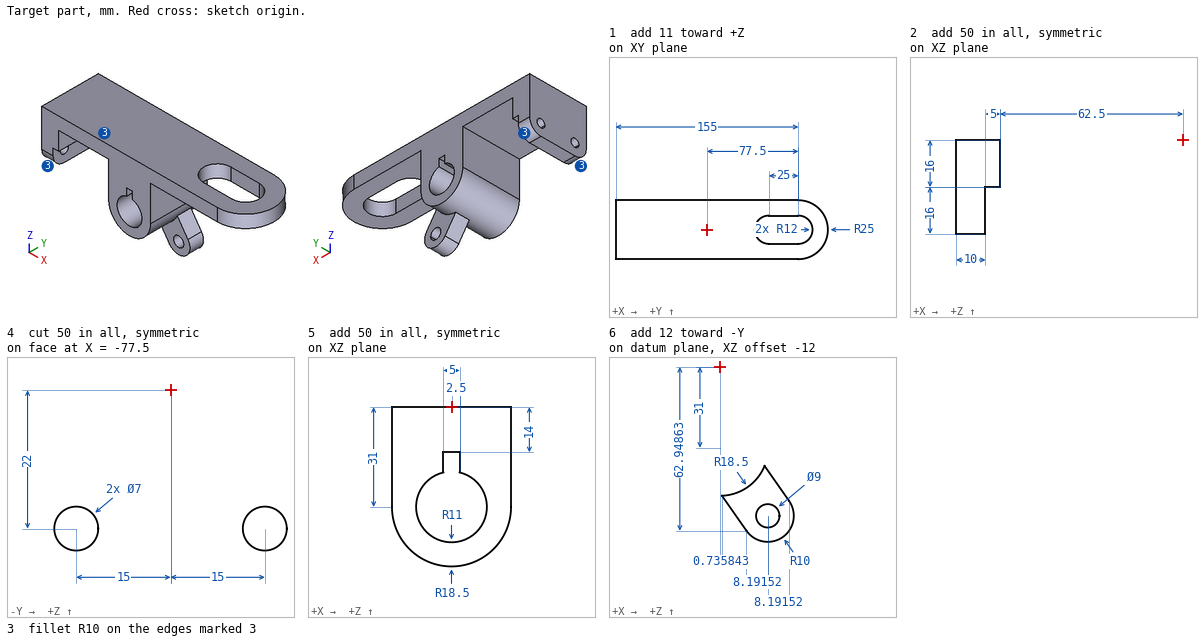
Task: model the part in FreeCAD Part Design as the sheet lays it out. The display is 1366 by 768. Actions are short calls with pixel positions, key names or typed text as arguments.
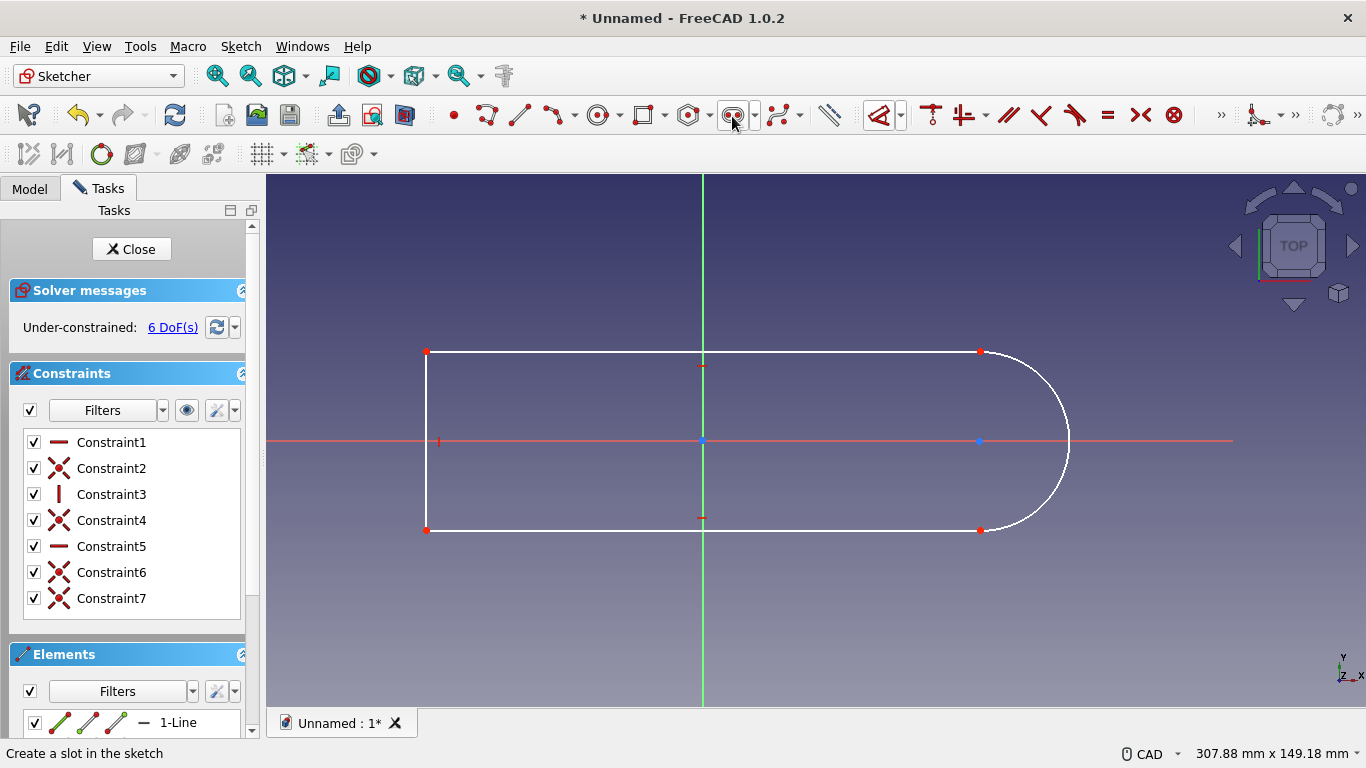
click(891, 440)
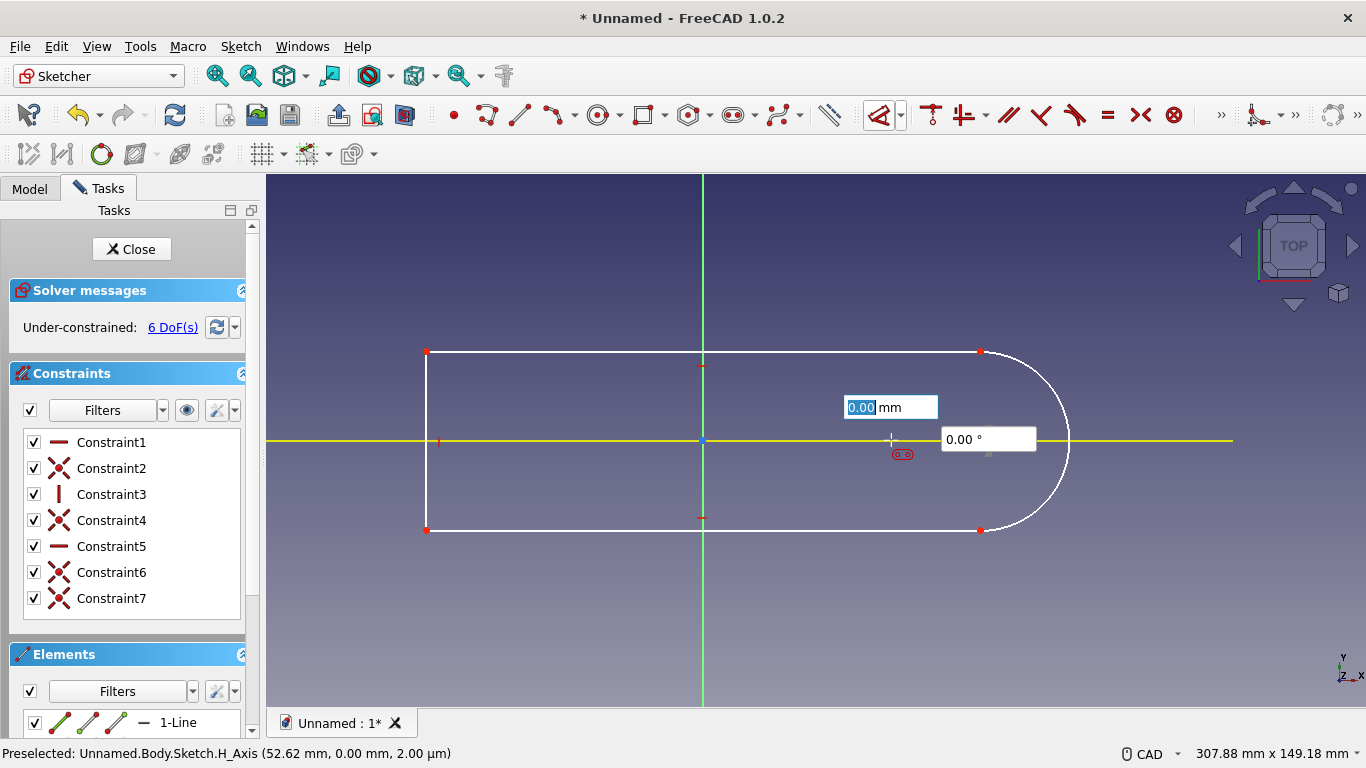
click(980, 432)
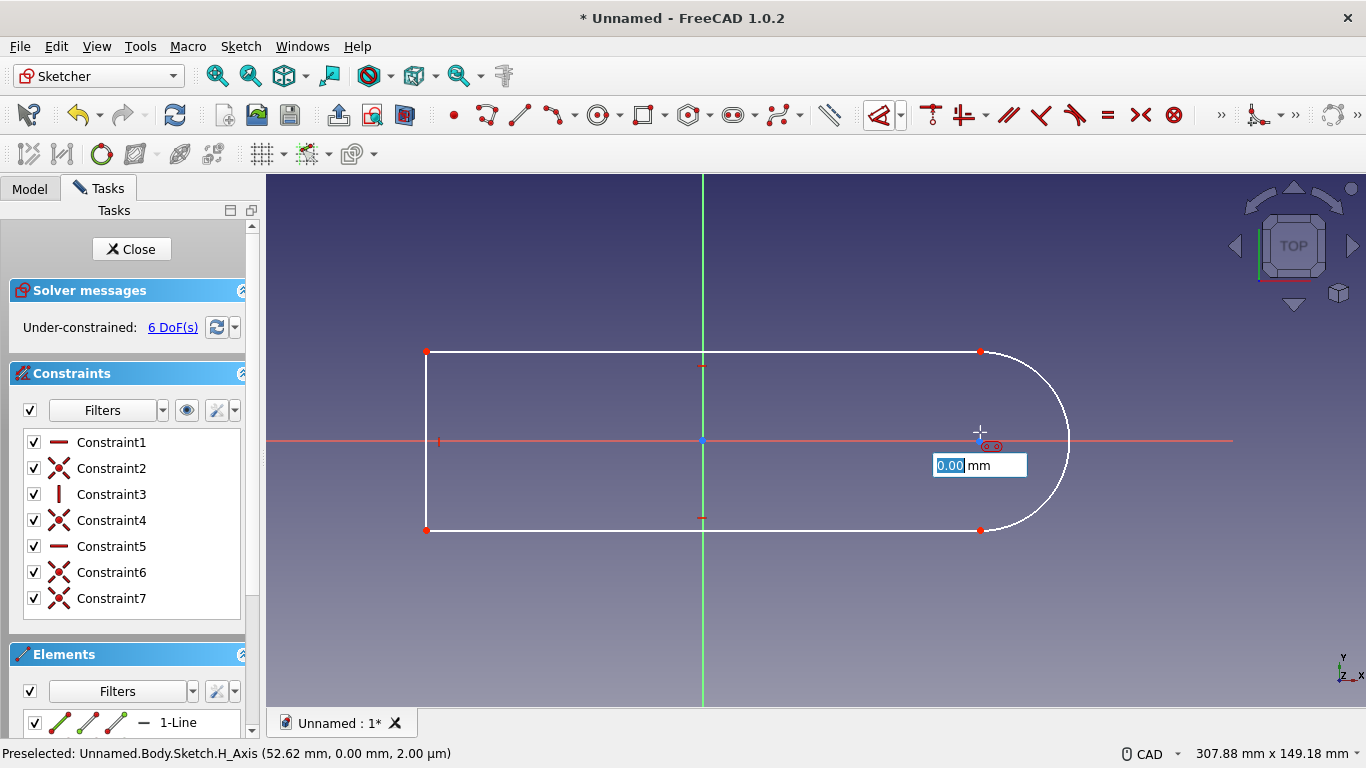
click(935, 398)
key(Escape)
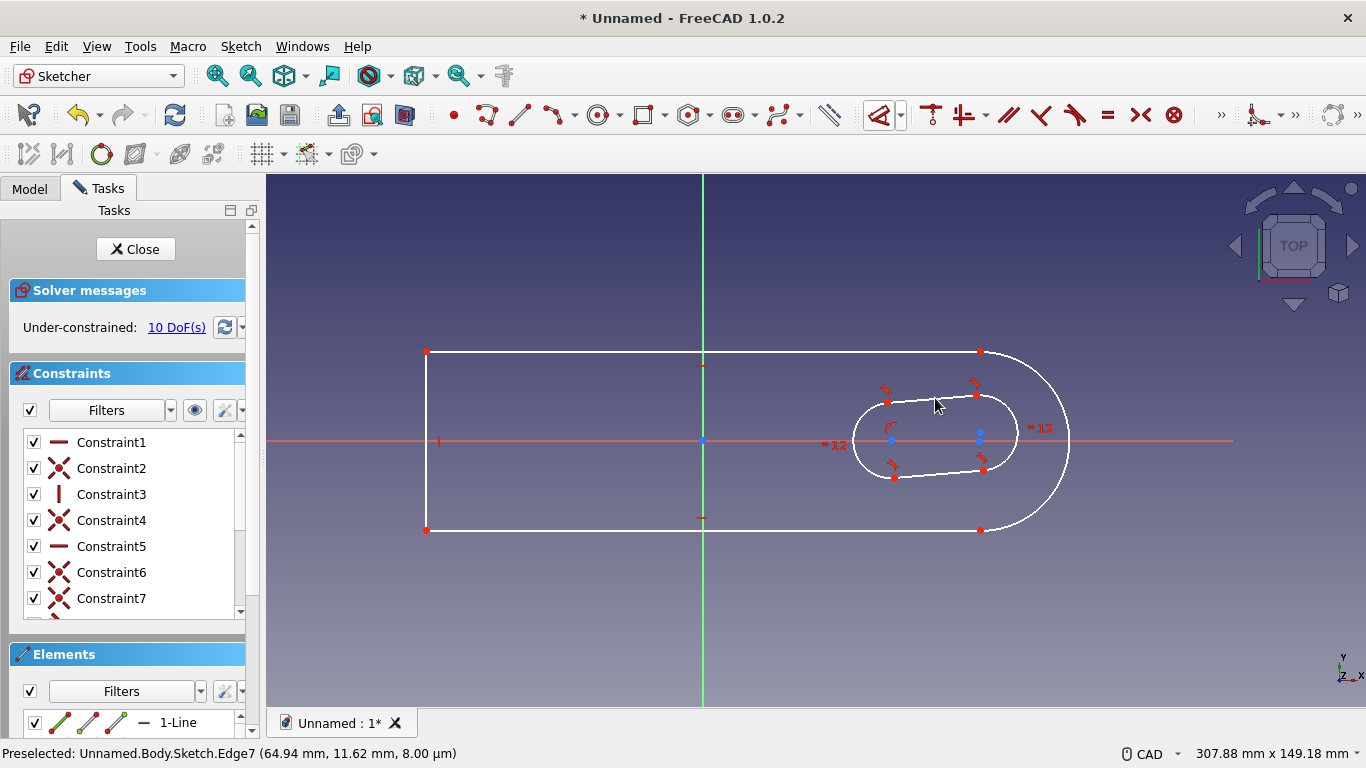
click(814, 352)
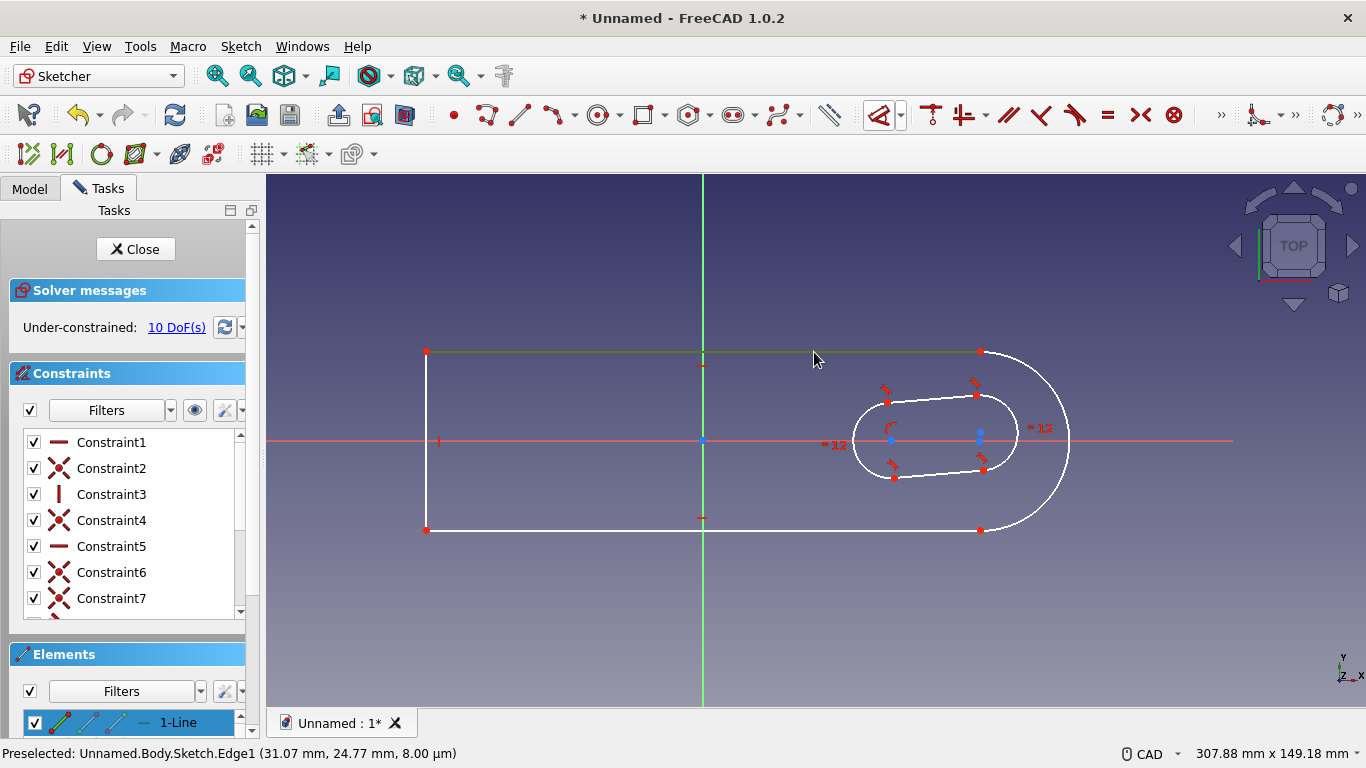
click(1052, 494)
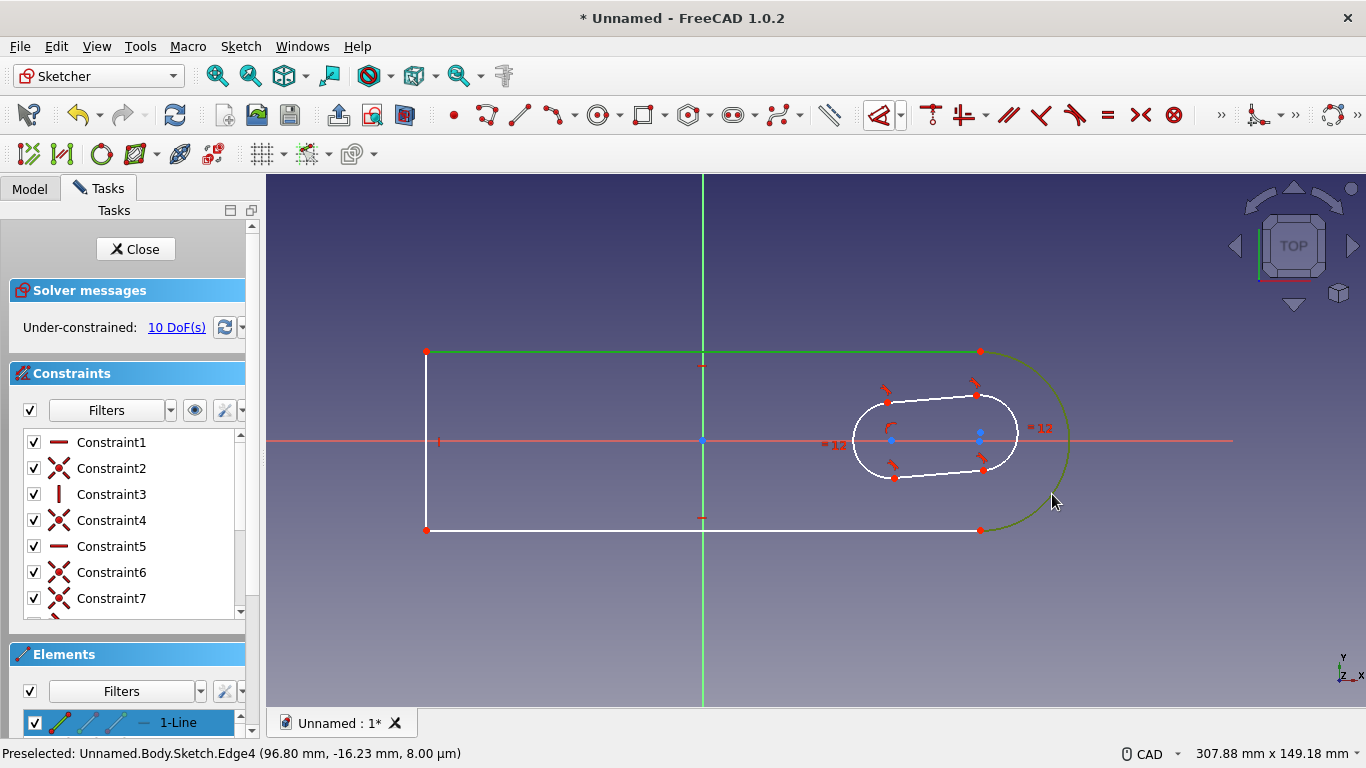
key(t)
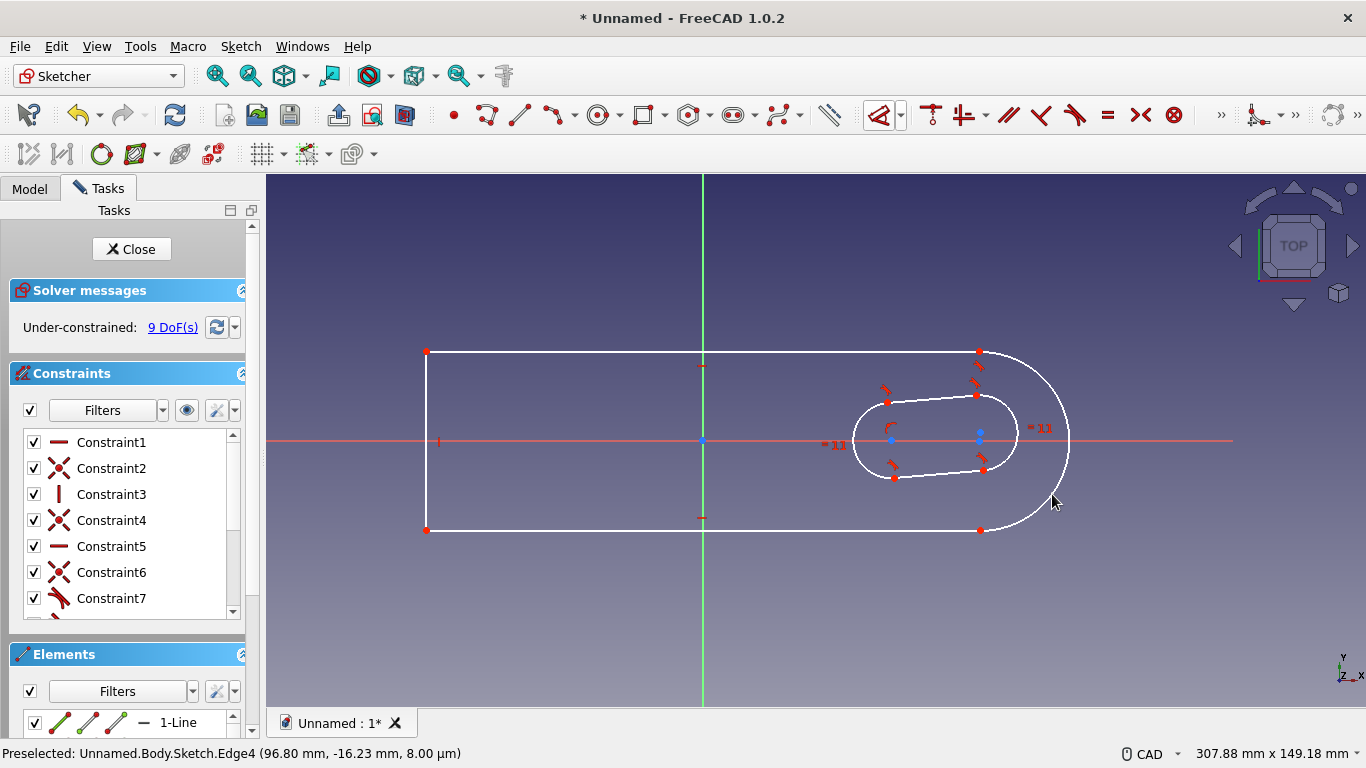
click(592, 531)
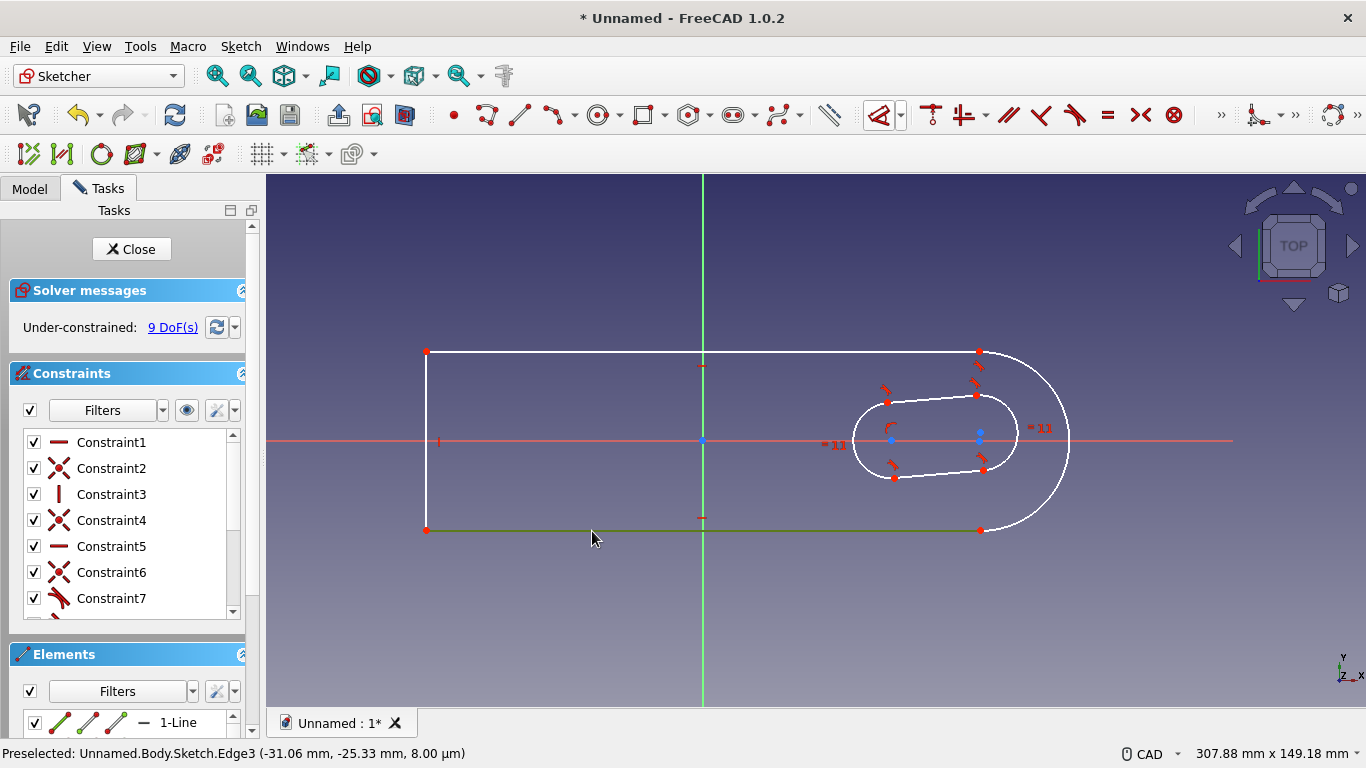
click(1052, 494)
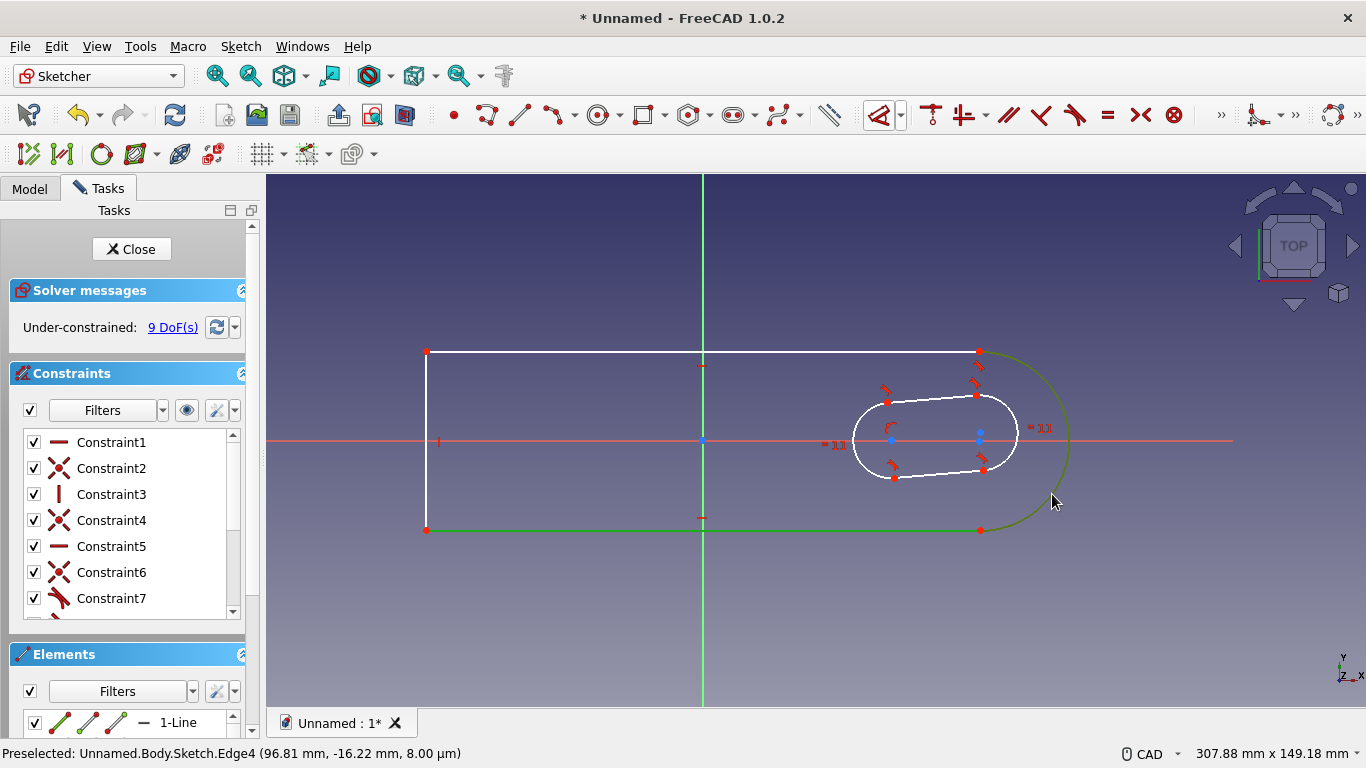
click(1075, 116)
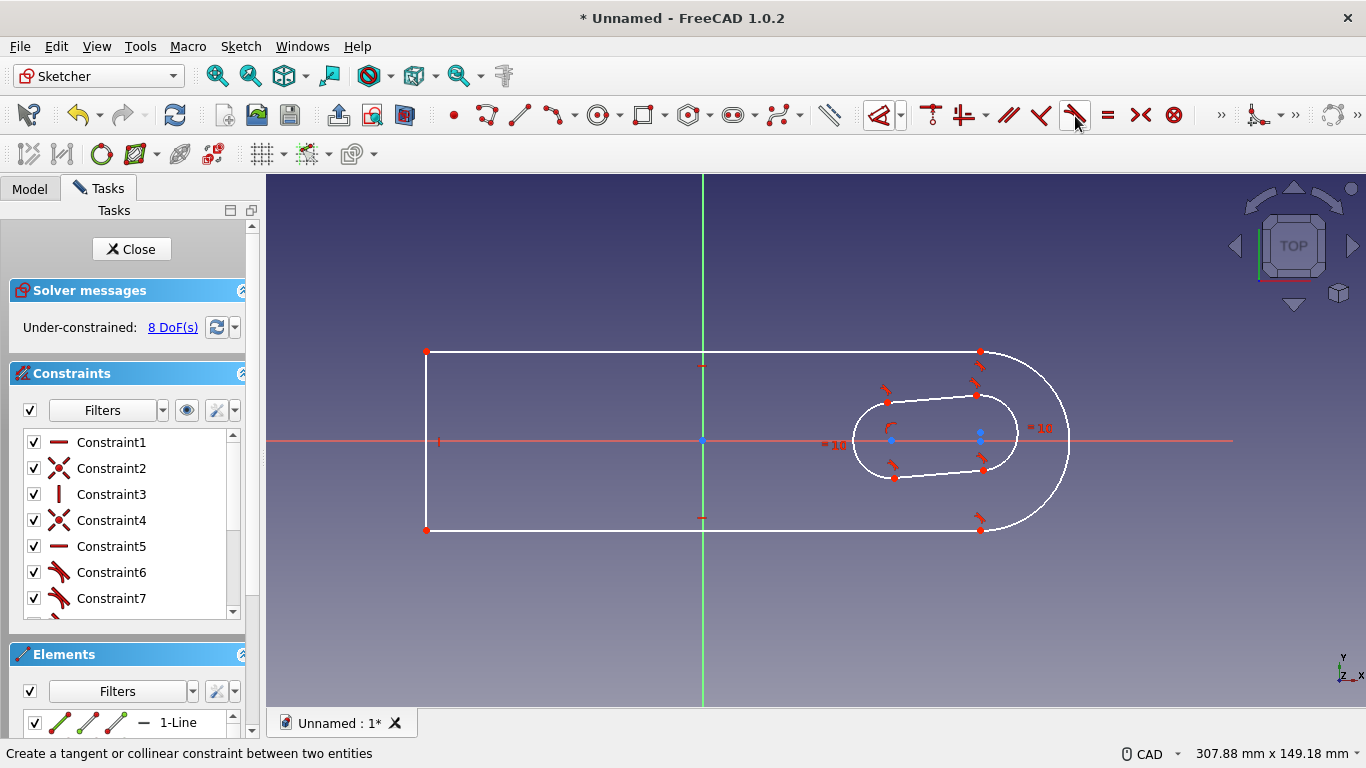
click(915, 401)